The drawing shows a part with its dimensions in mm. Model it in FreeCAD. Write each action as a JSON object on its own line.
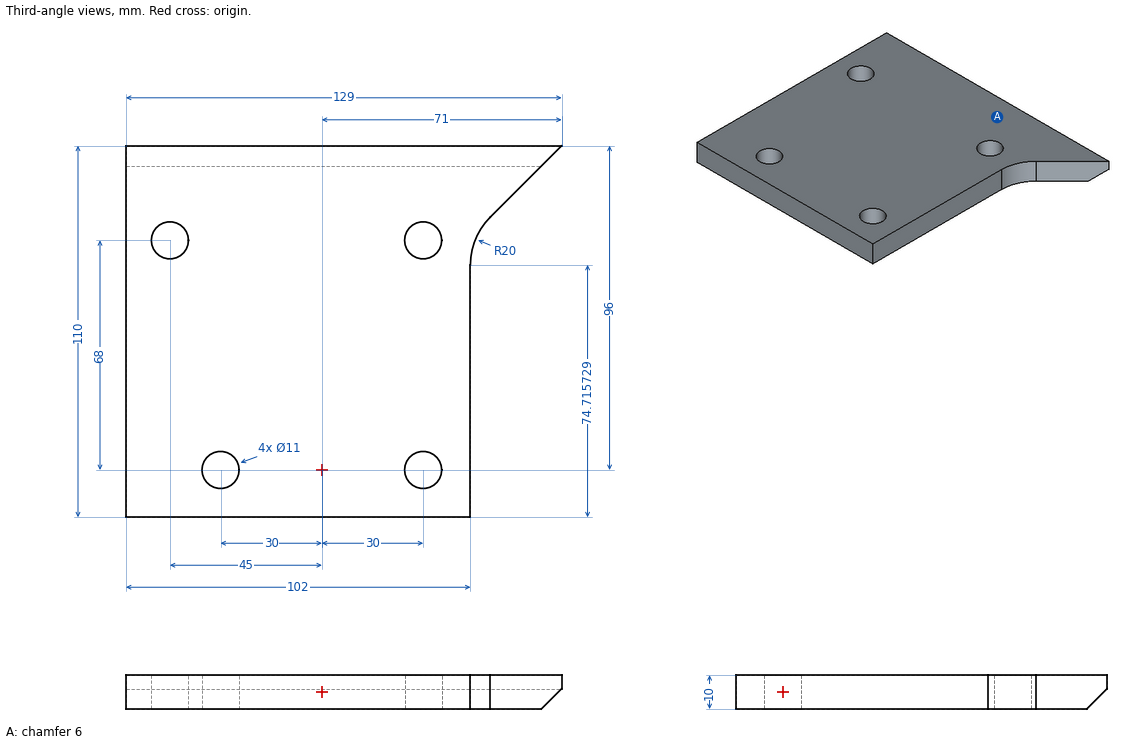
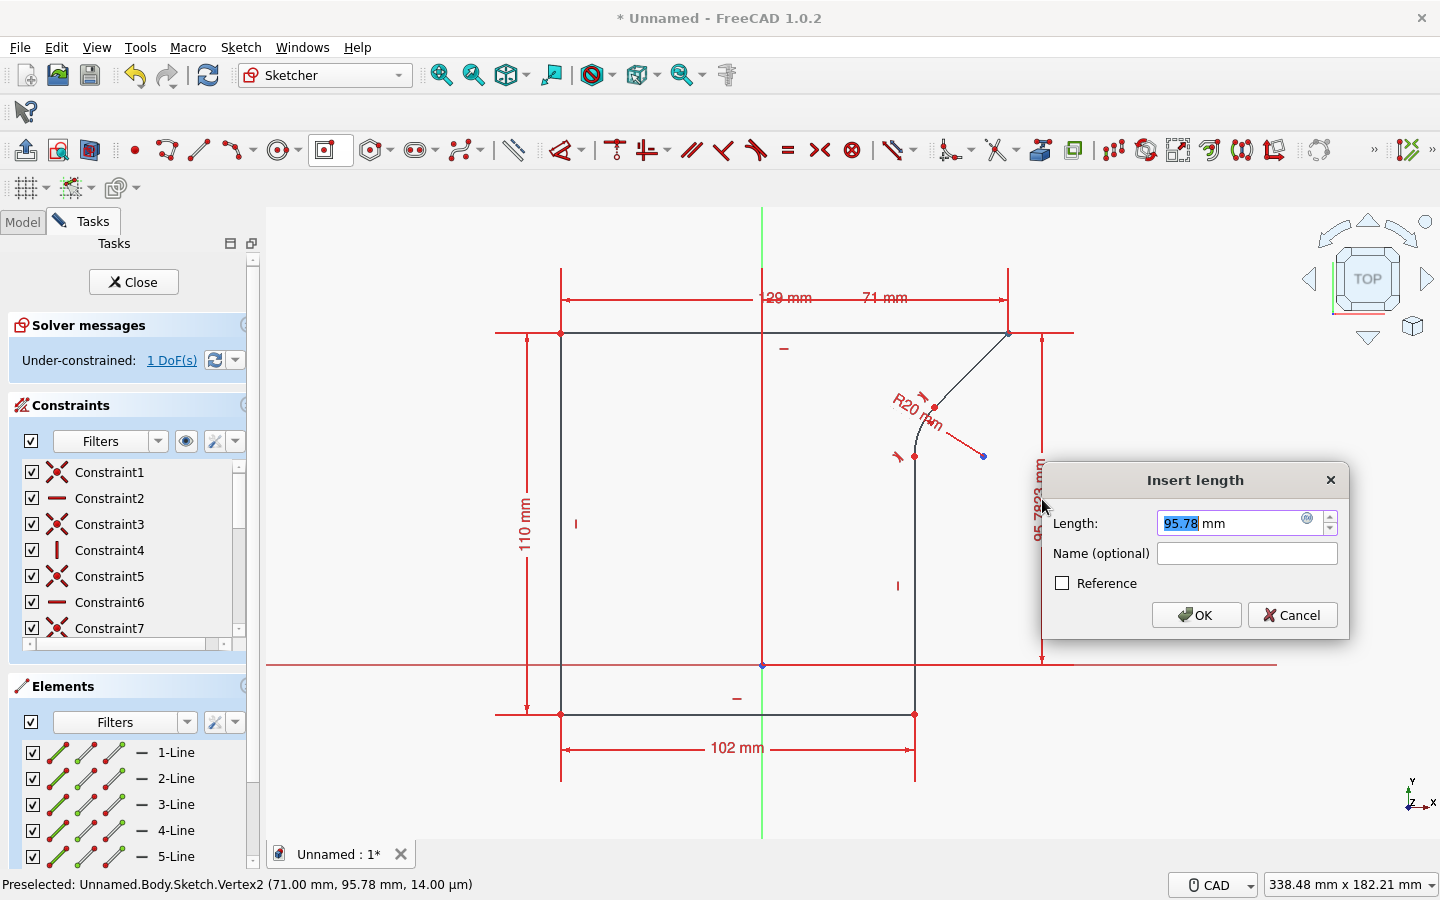
{"action": "type", "text": "96"}
{"action": "key", "text": "Return"}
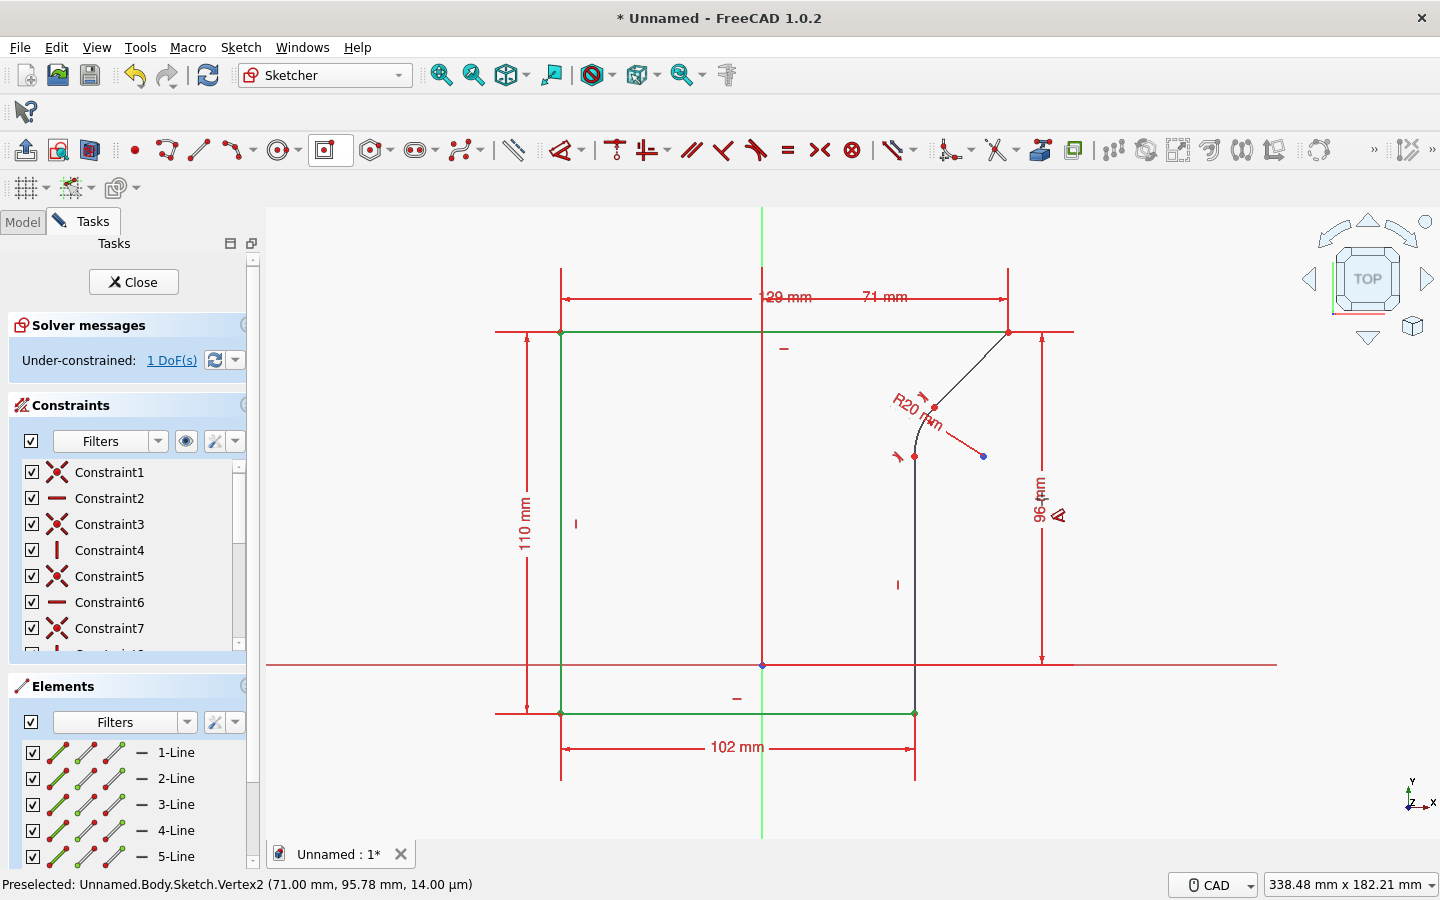
{"action": "left_click", "coordinate": [915, 636]}
{"action": "left_click", "coordinate": [949, 585]}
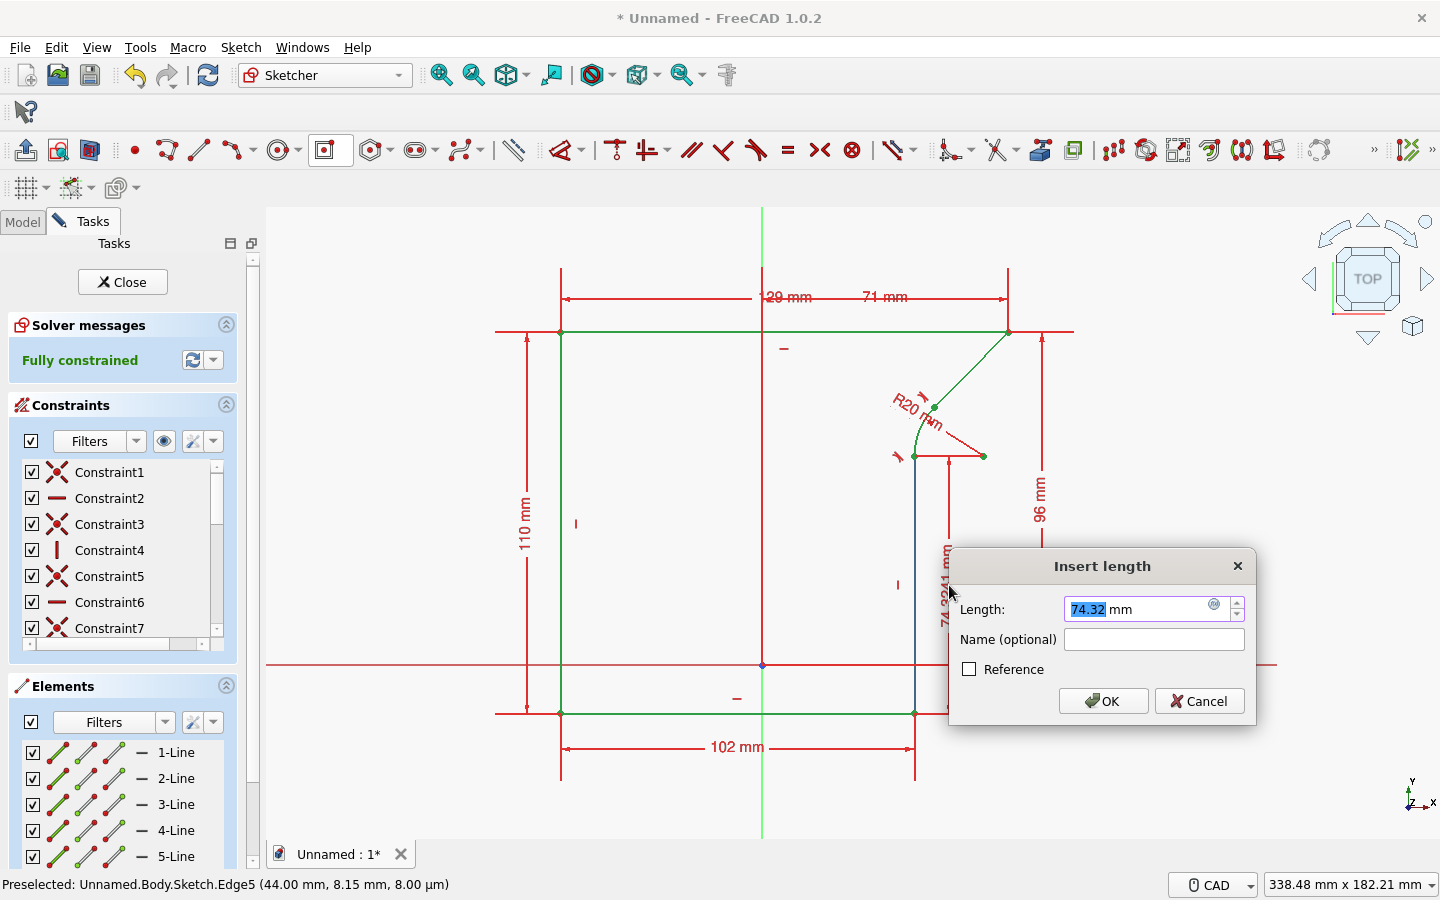
{"action": "type", "text": "74.715729"}
{"action": "key", "text": "Return"}
{"action": "key", "text": "Escape"}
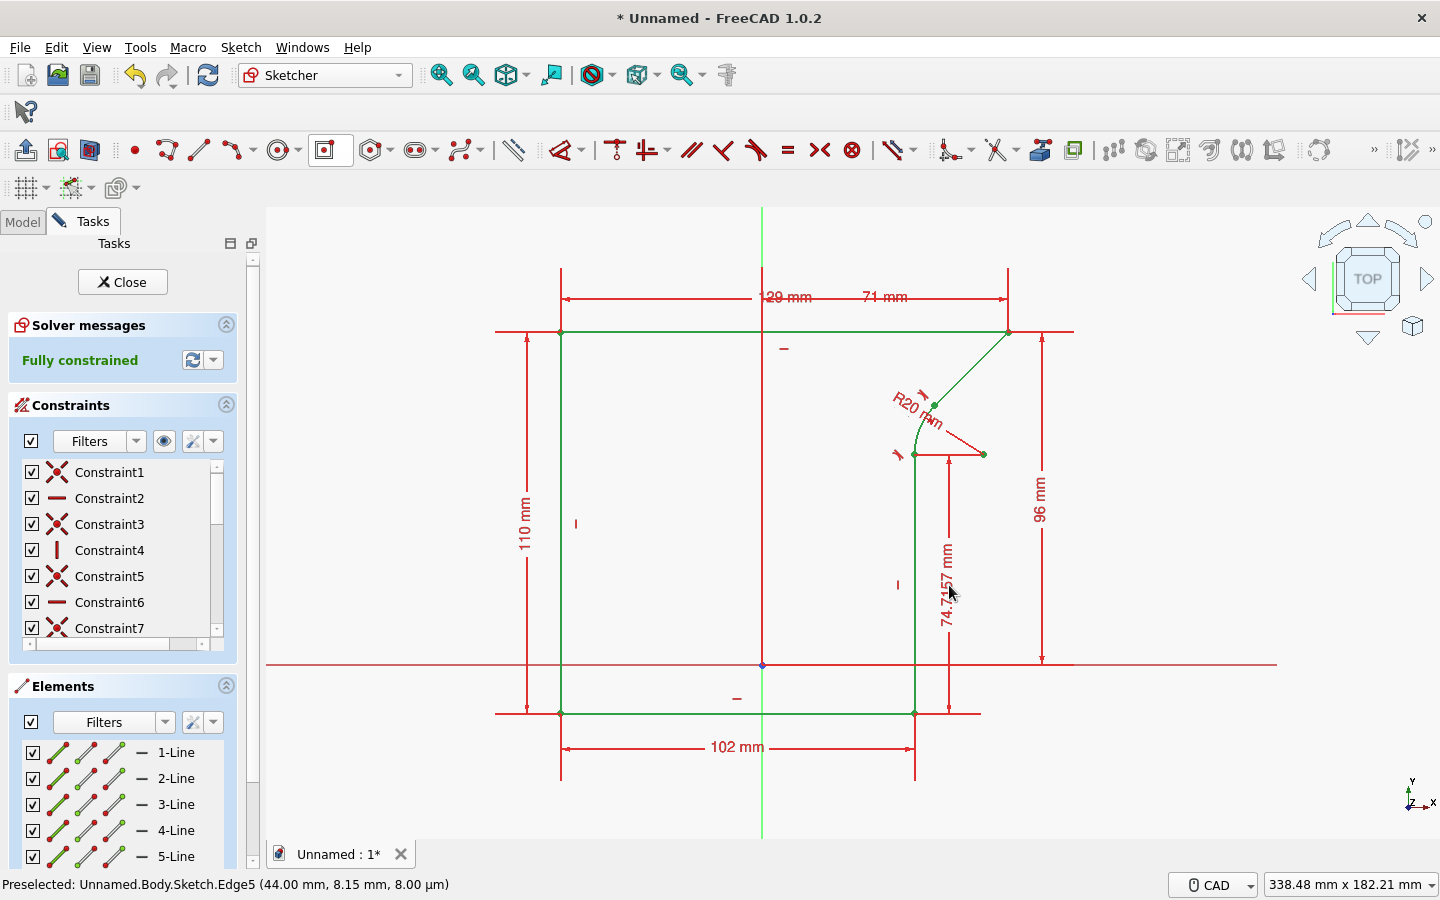
{"action": "left_click", "coordinate": [123, 282]}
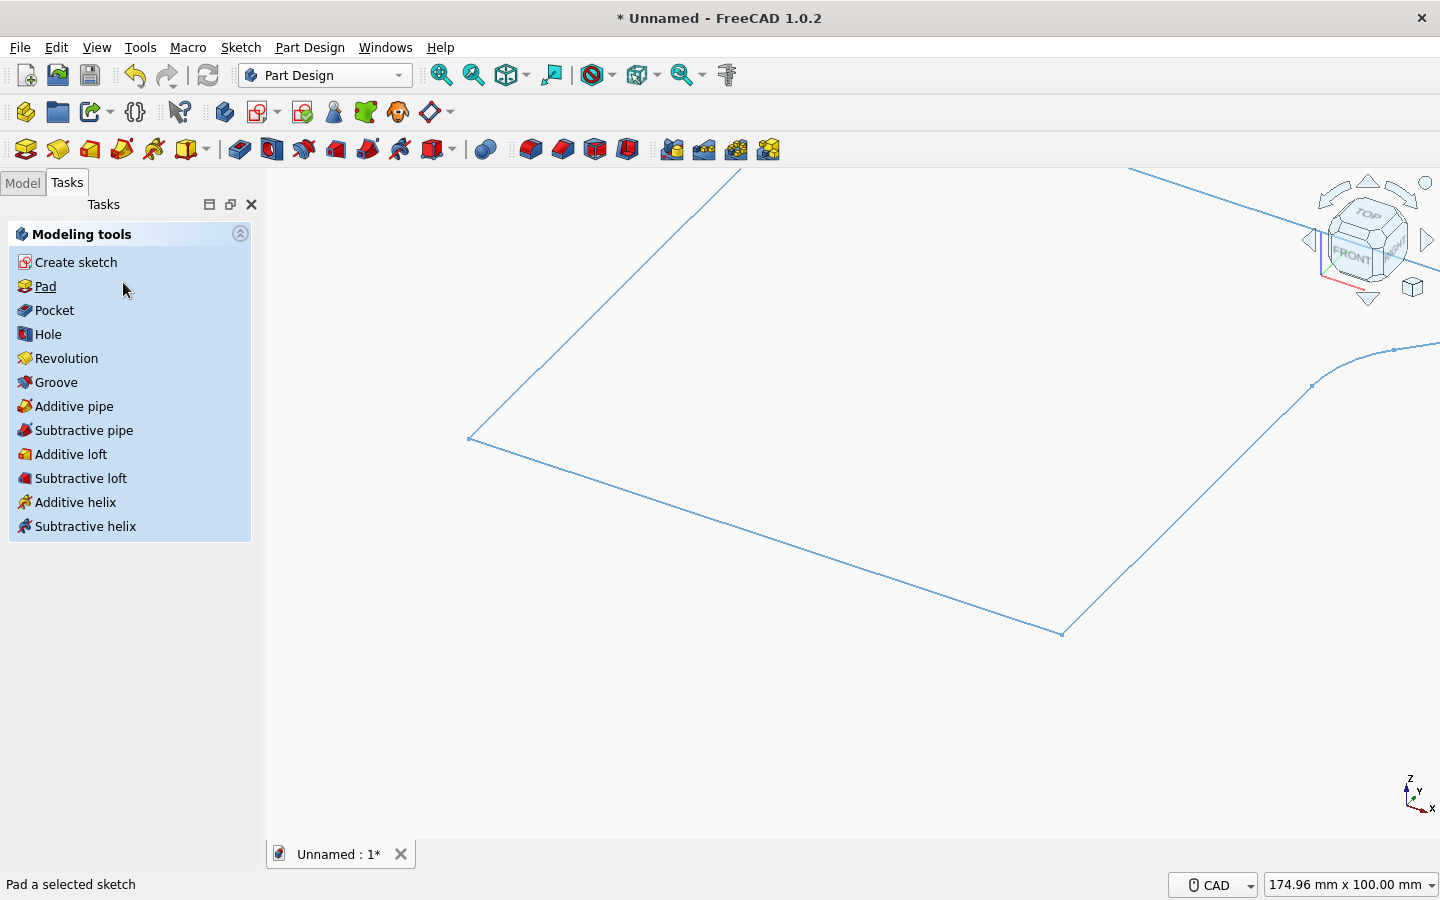
{"action": "left_click", "coordinate": [26, 150]}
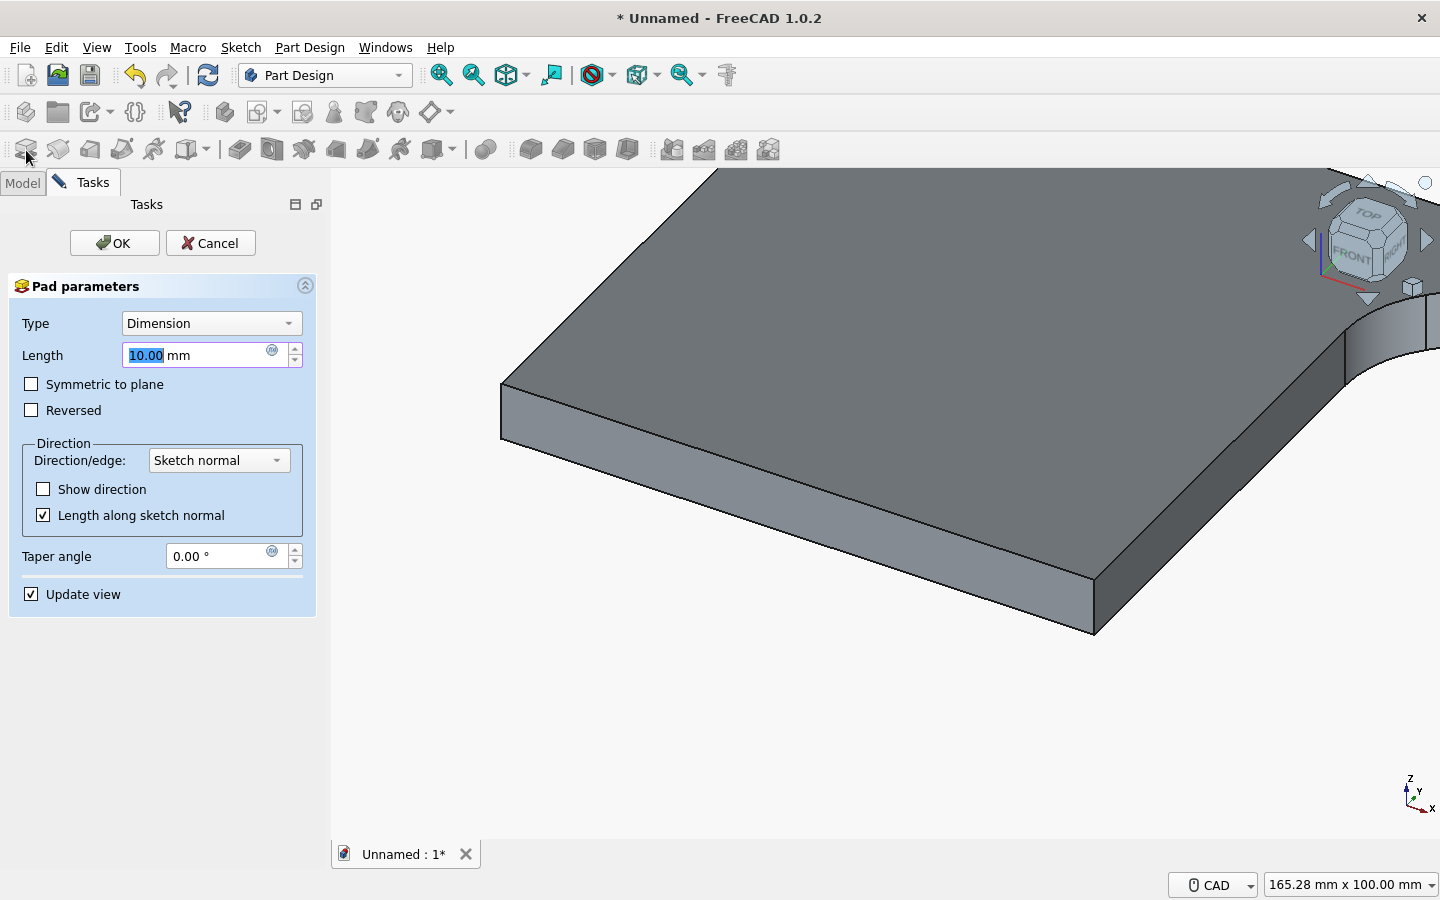
{"action": "type", "text": "10"}
{"action": "key", "text": "Tab"}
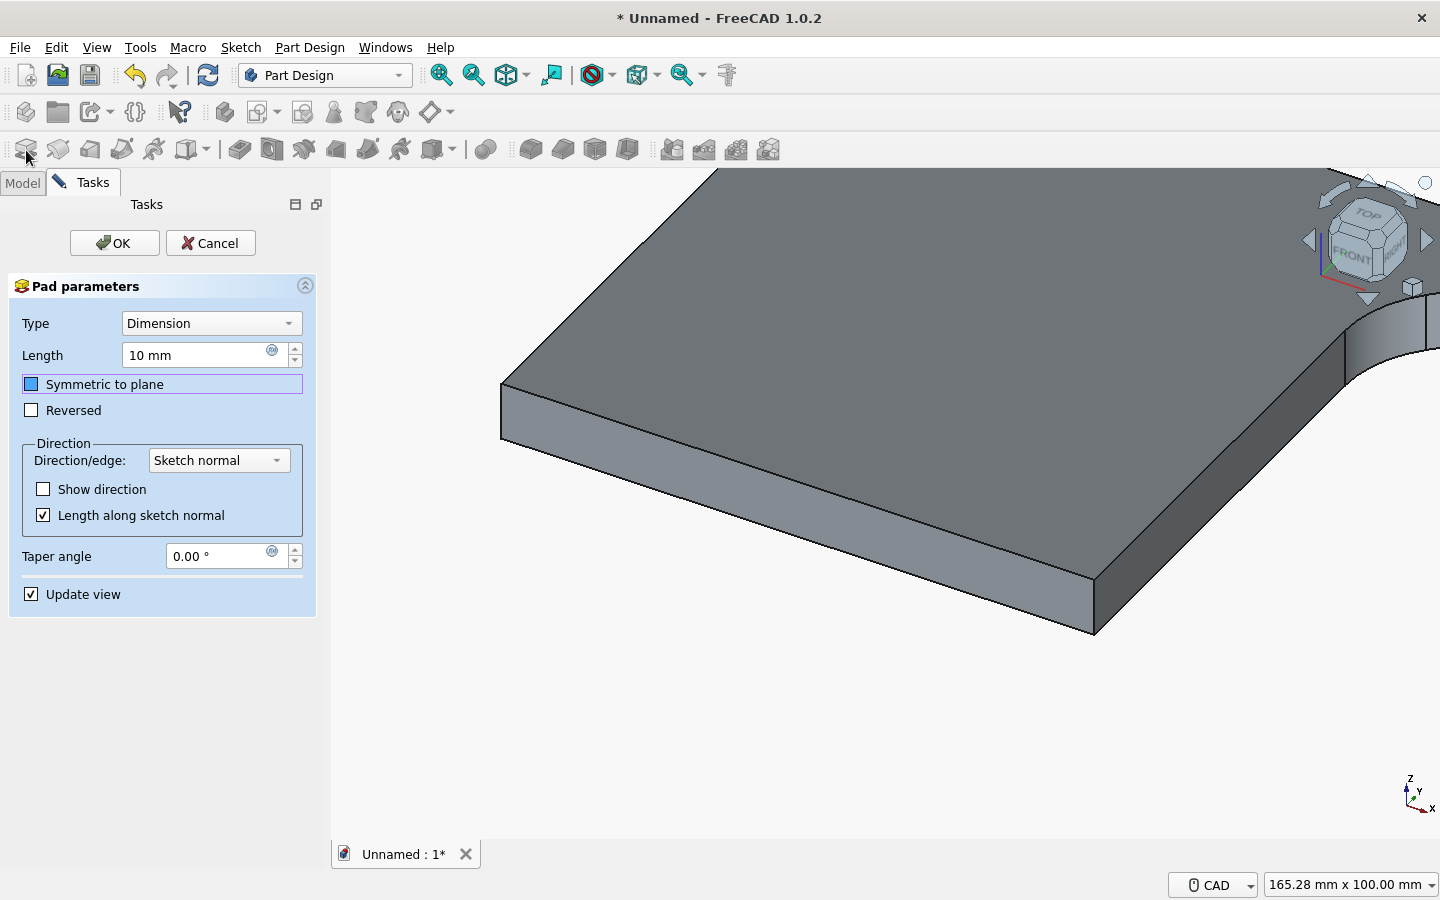
{"action": "left_click", "coordinate": [30, 384]}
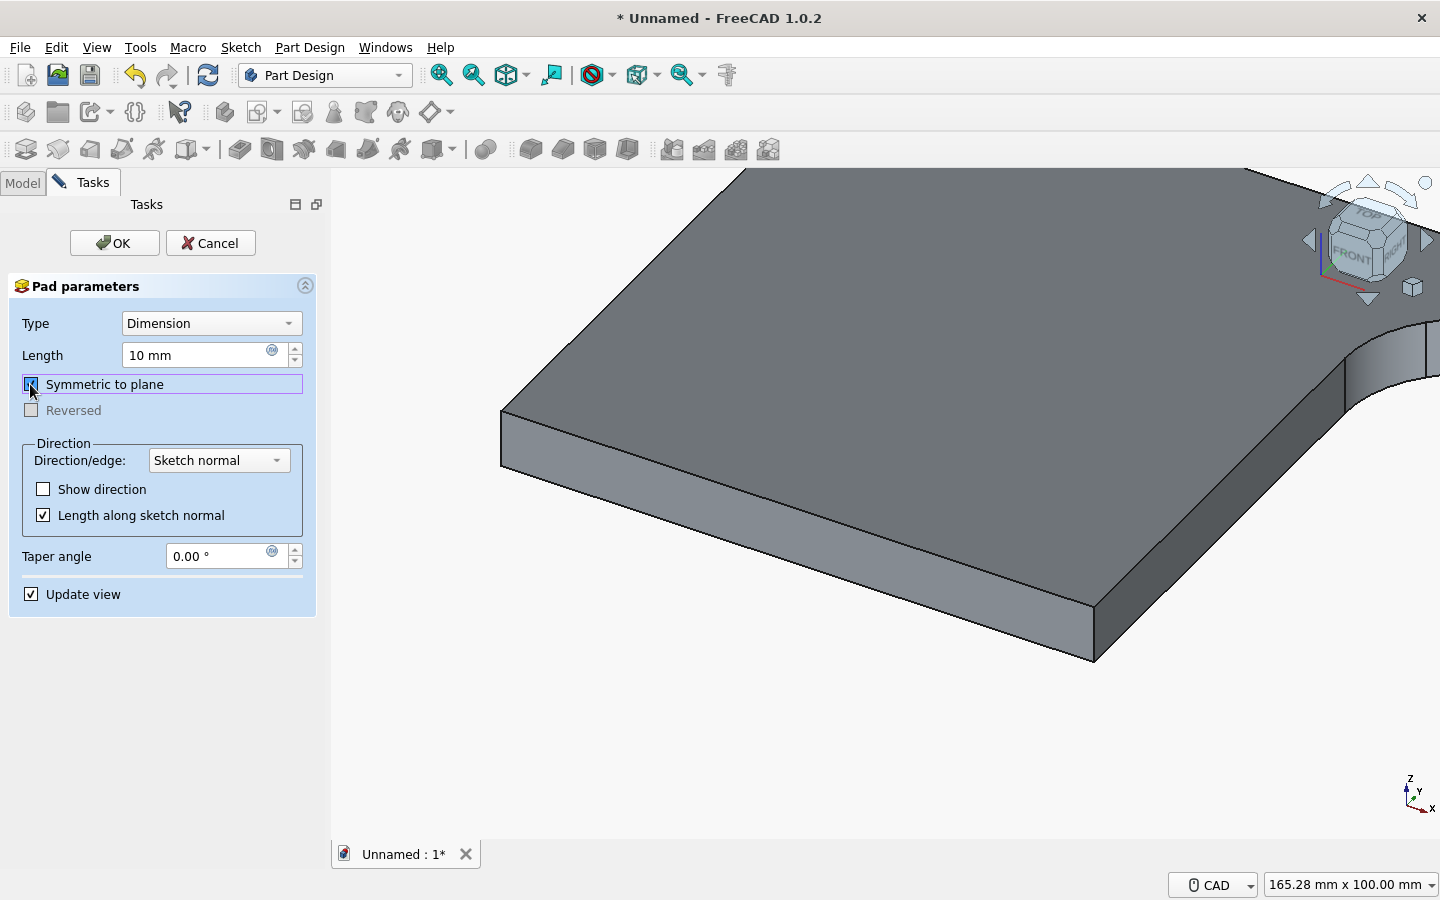
{"action": "left_click", "coordinate": [115, 243]}